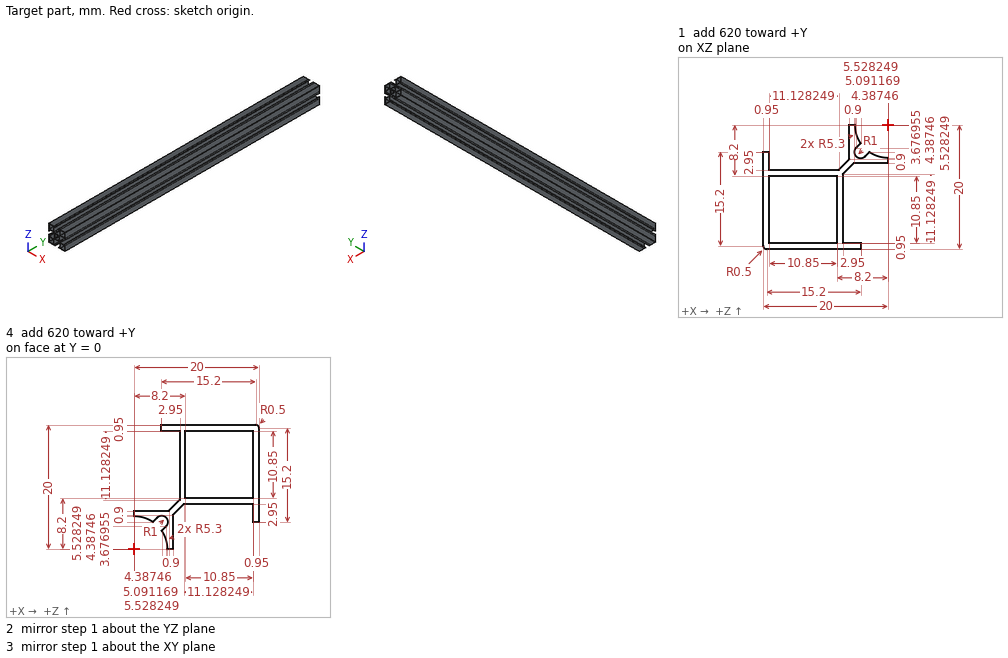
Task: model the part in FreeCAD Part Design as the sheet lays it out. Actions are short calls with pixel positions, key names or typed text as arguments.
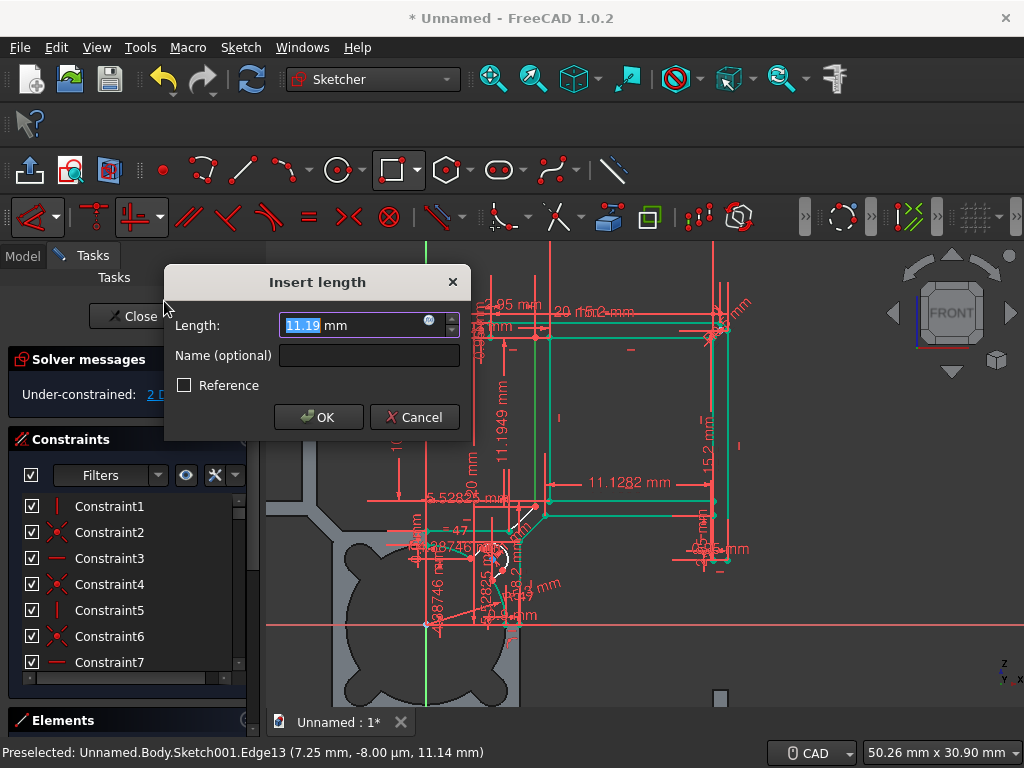
text(11.128249)
key(Return)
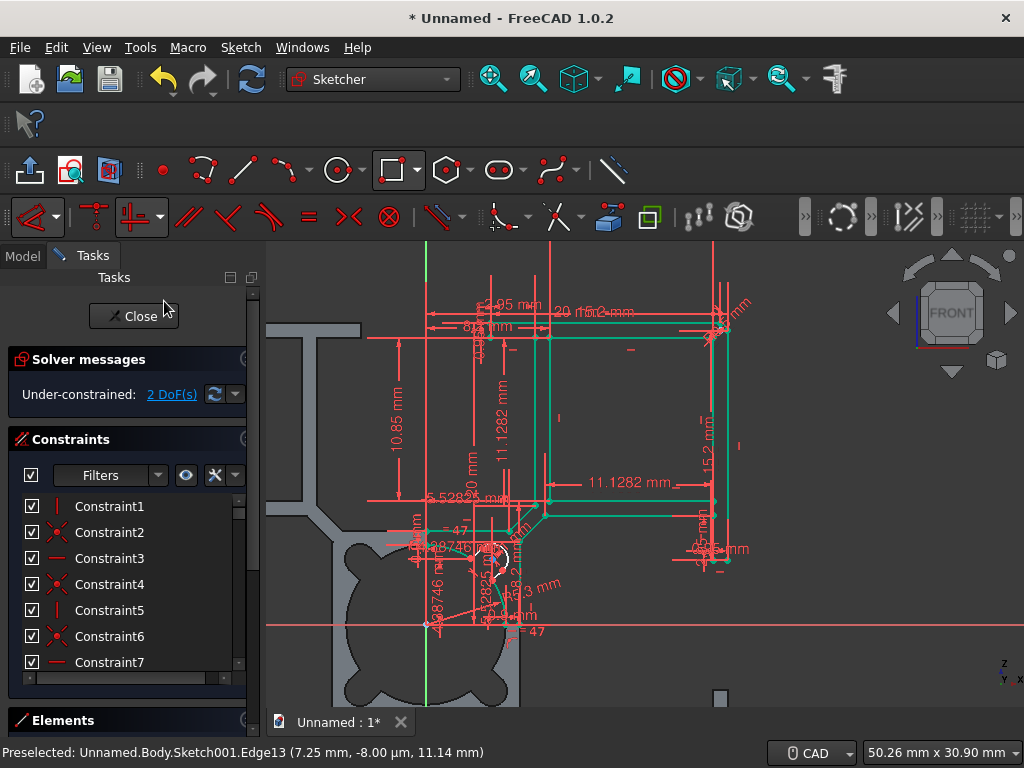
click(503, 571)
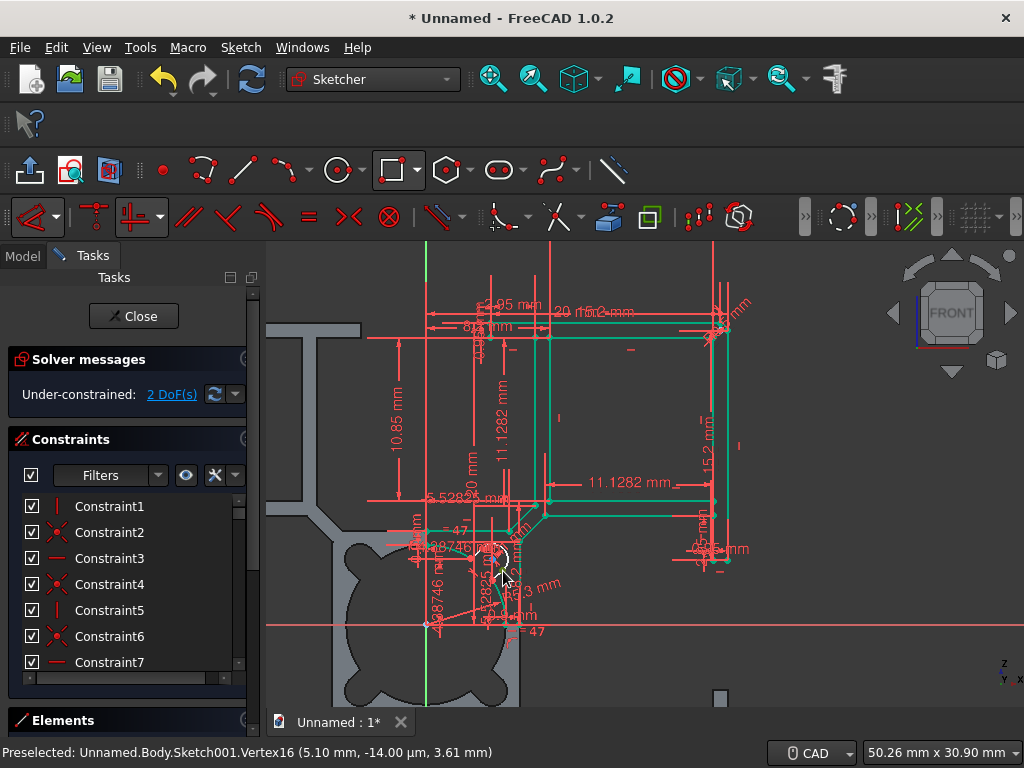
click(58, 218)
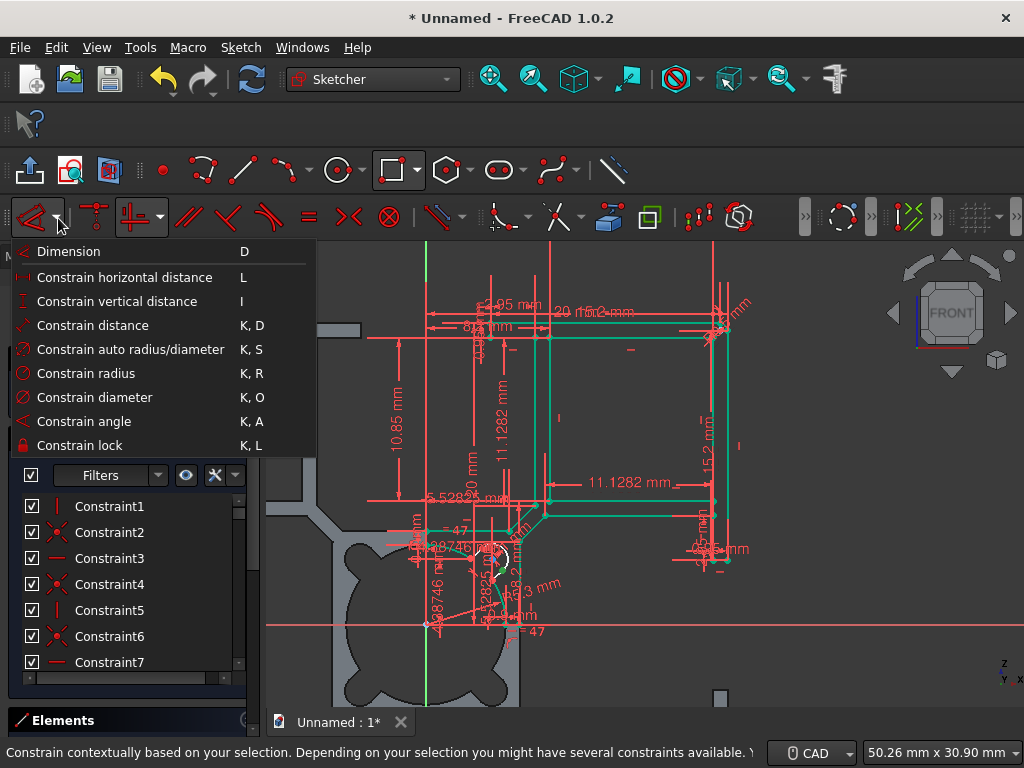
click(164, 277)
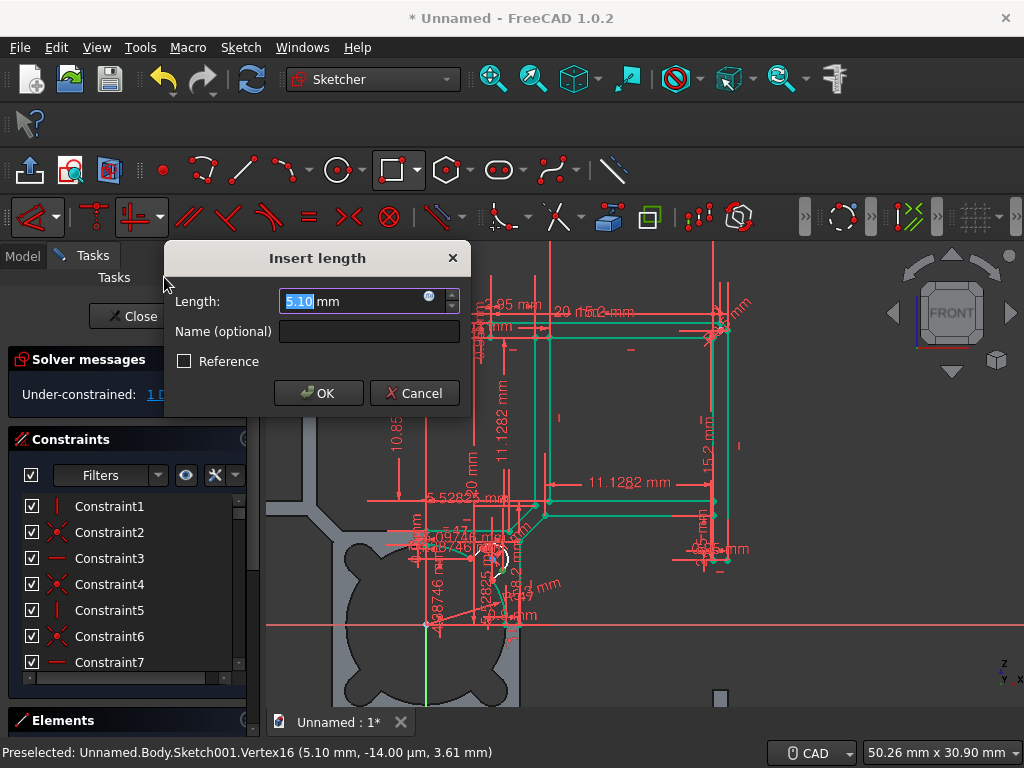
text(5.091169)
key(Return)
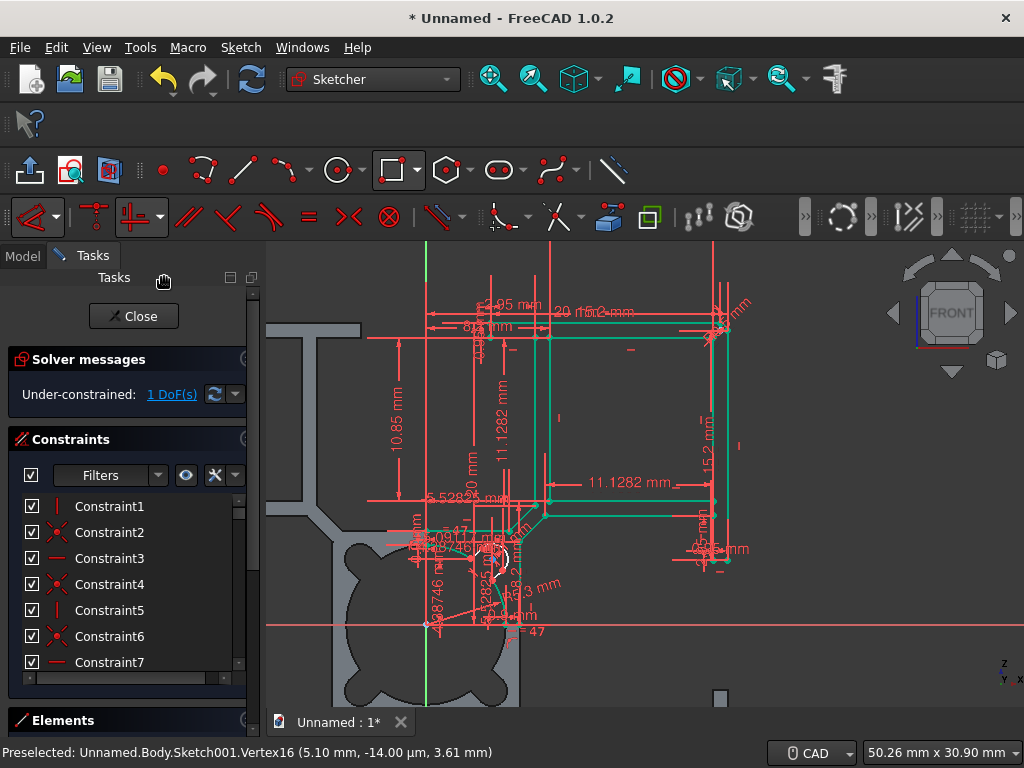
click(503, 571)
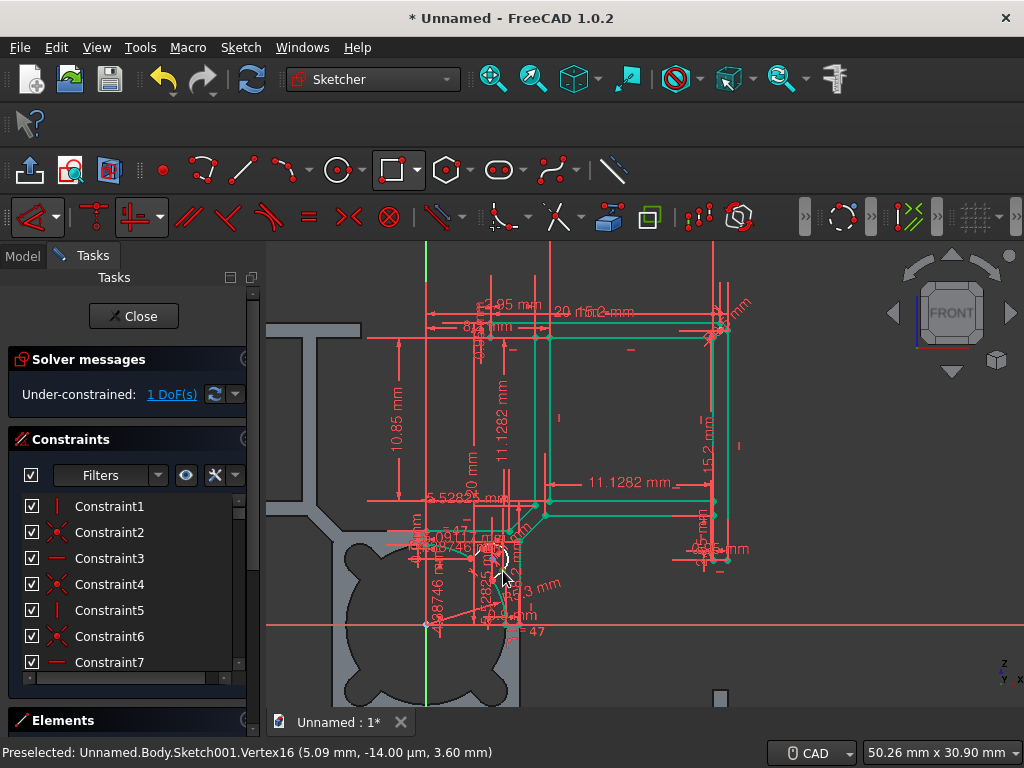
click(58, 218)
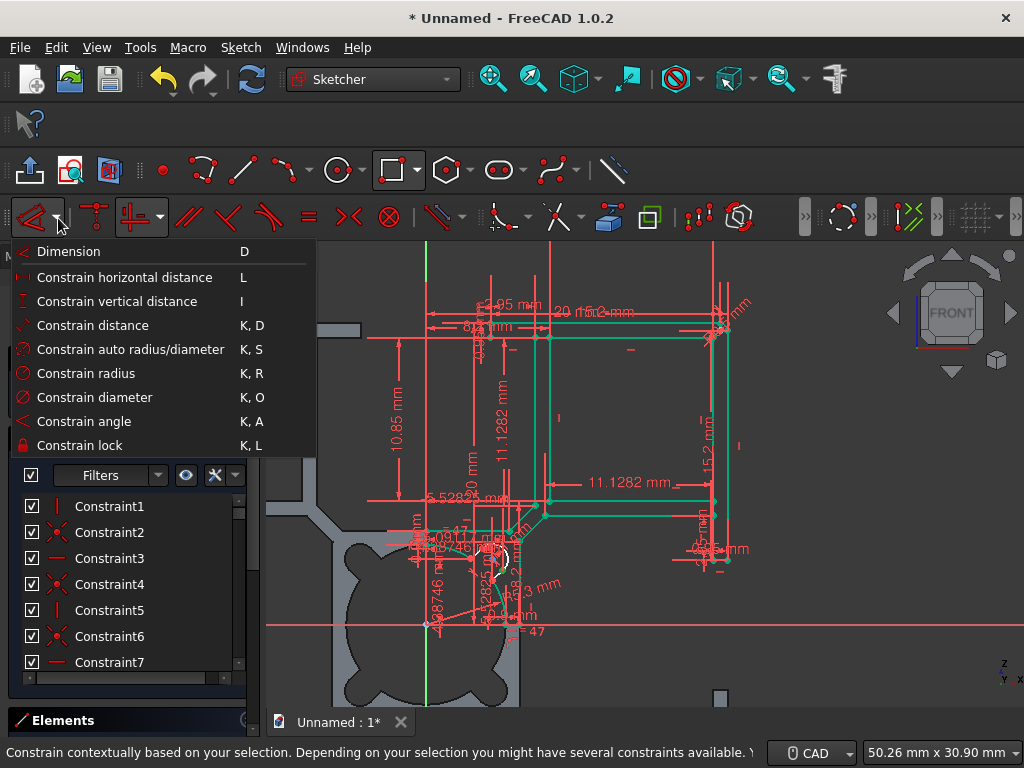
click(164, 301)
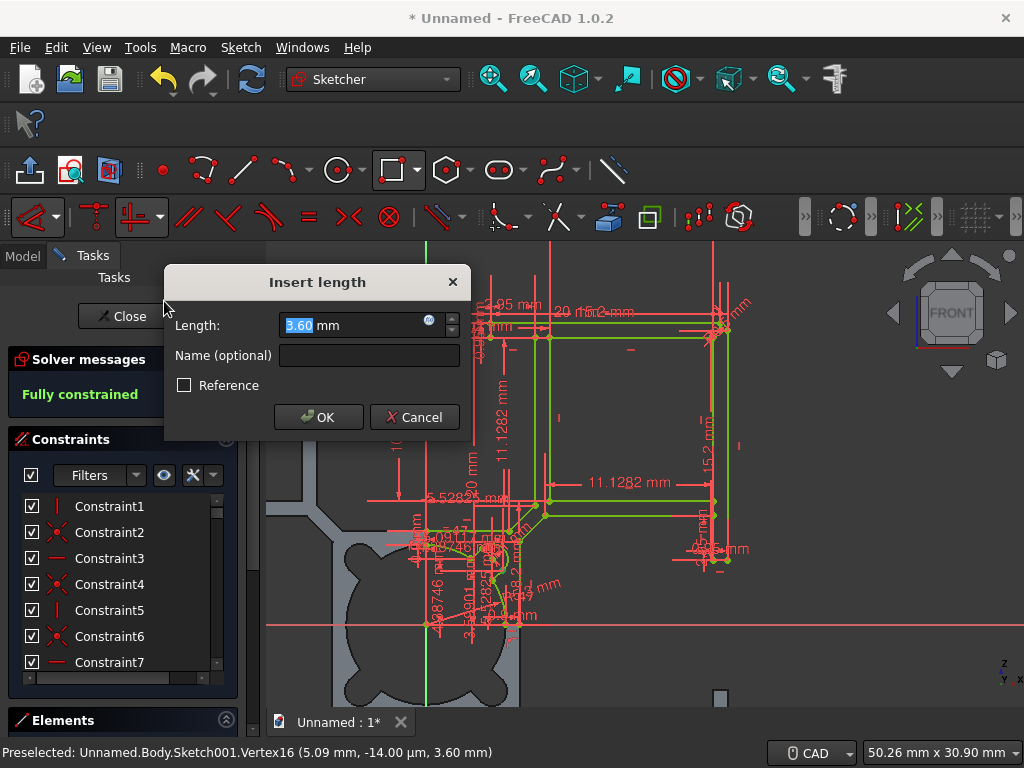
text(3.676955)
key(Return)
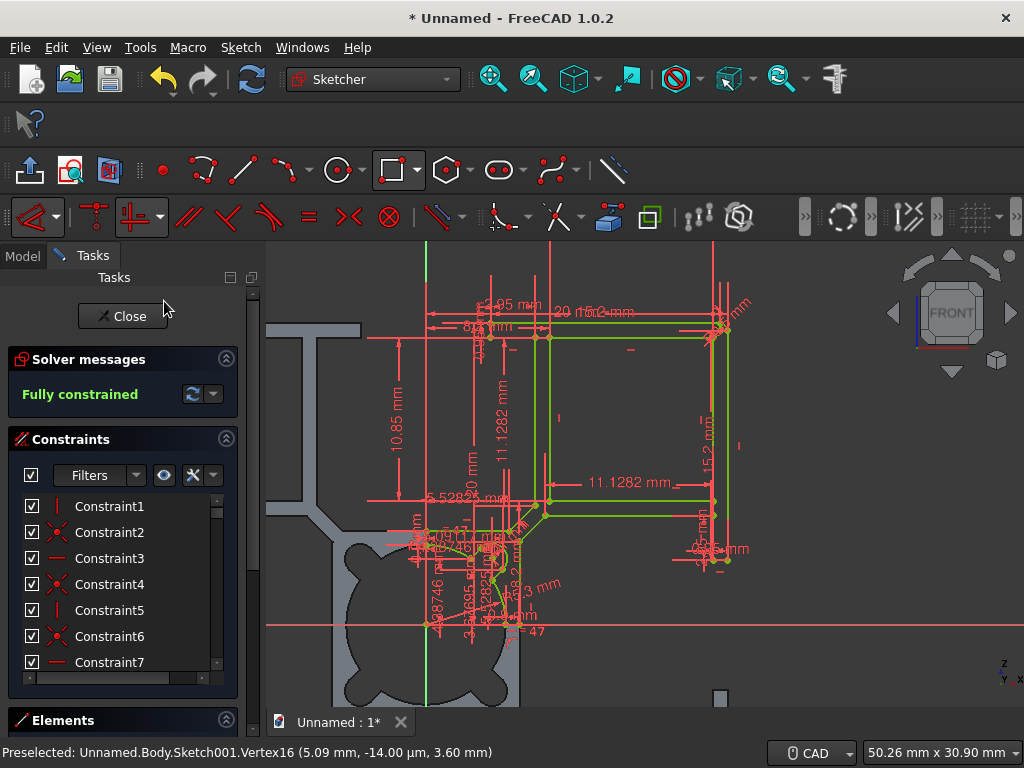
click(123, 316)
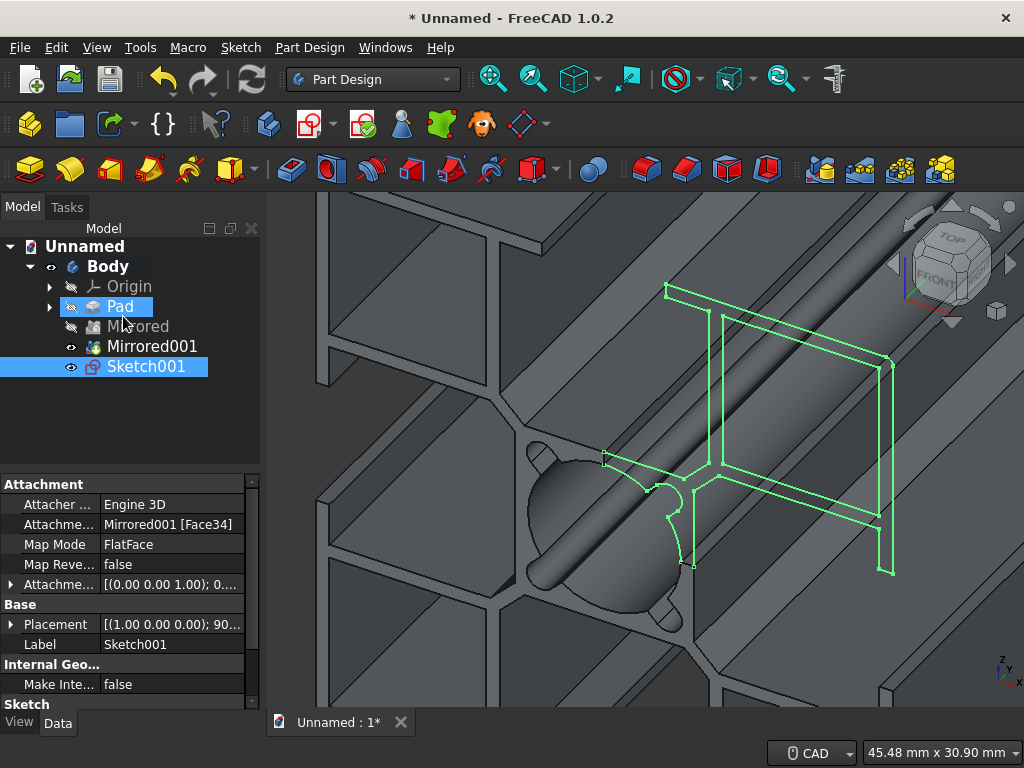
click(30, 170)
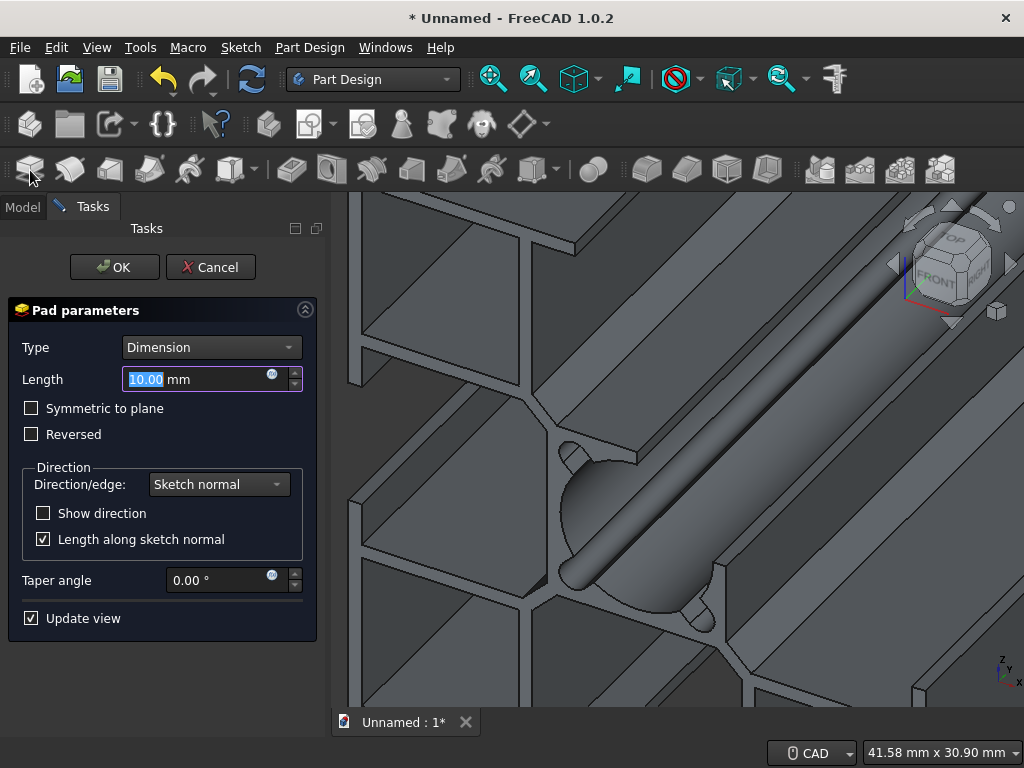
text(620)
key(Tab)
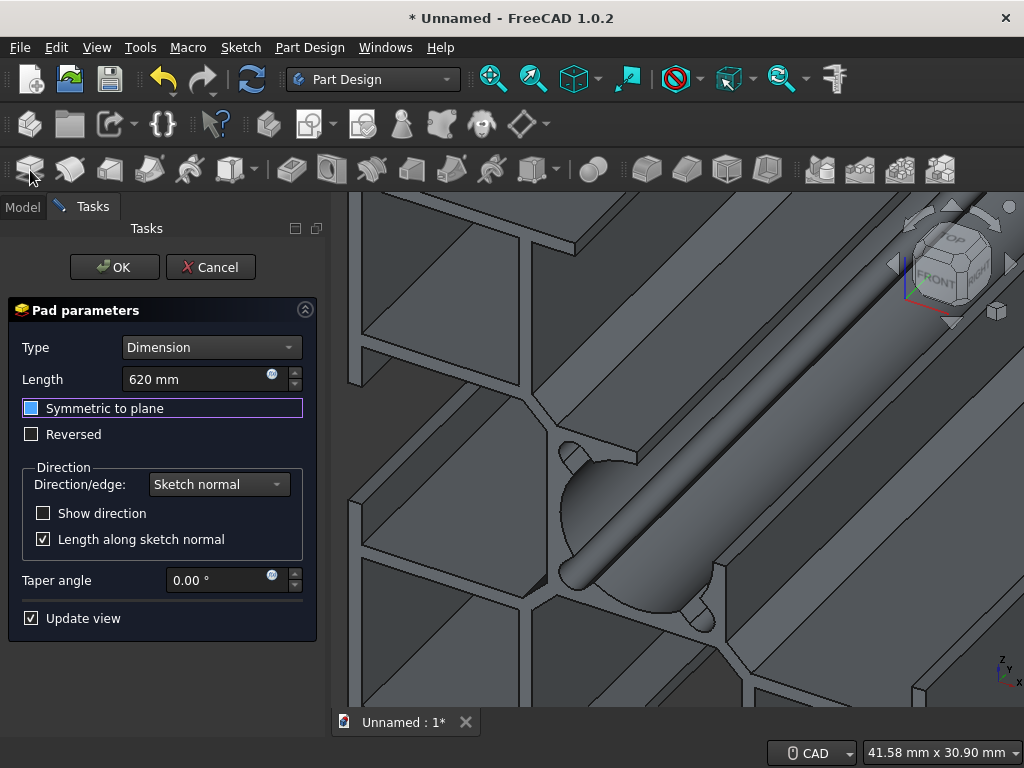
click(30, 434)